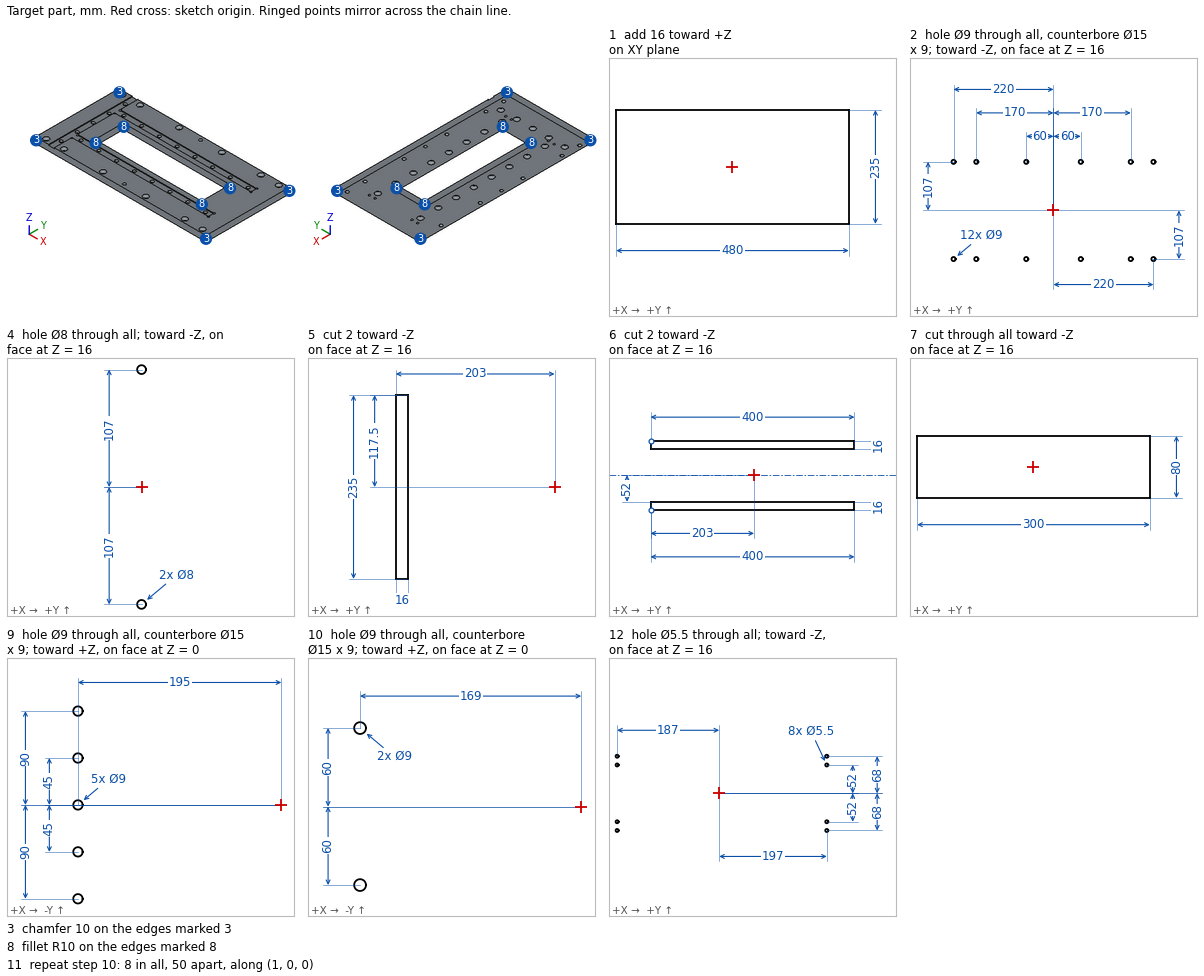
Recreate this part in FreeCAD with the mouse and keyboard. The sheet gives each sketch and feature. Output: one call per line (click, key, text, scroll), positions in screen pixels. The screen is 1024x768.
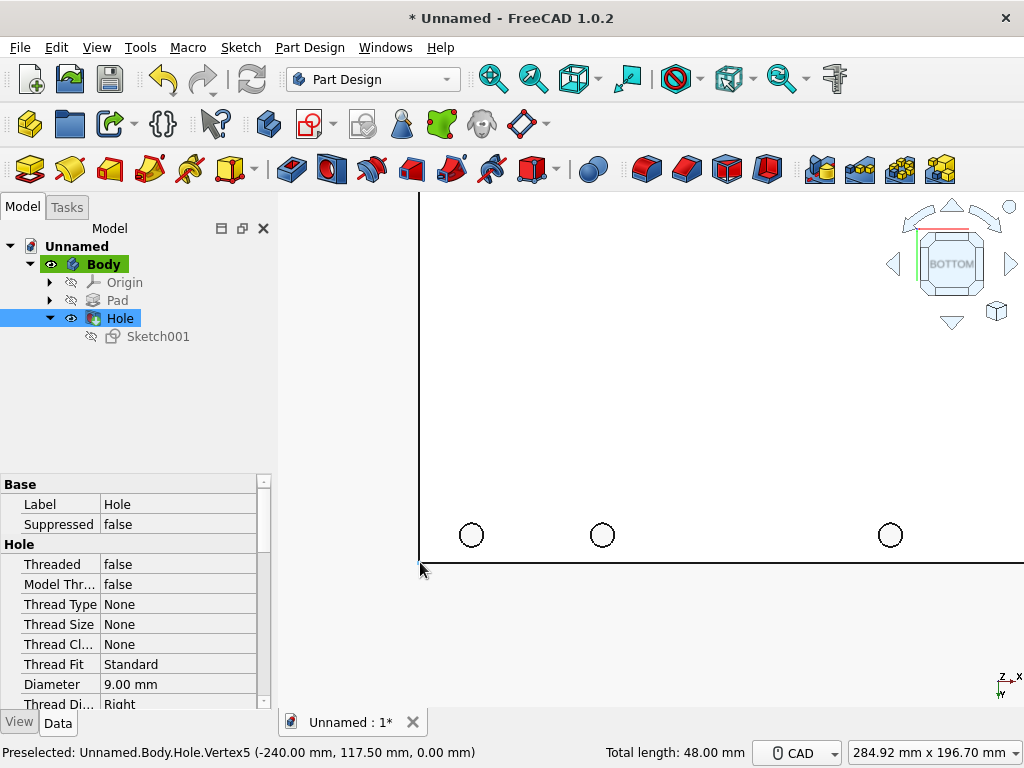
click(494, 80)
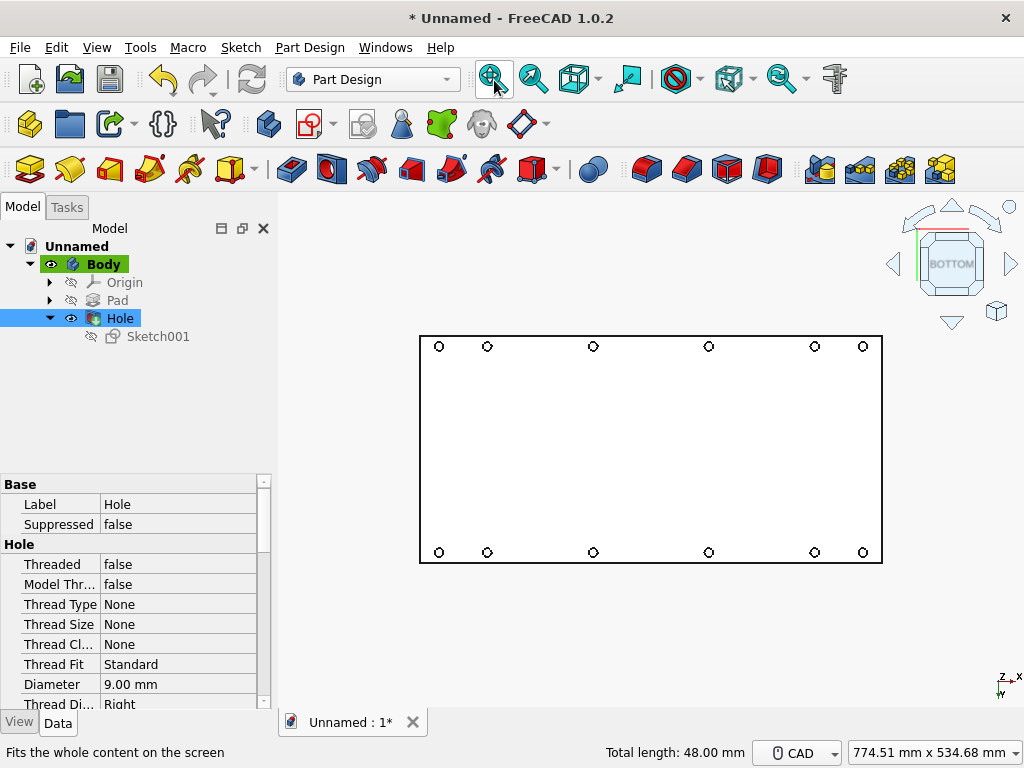
key(4)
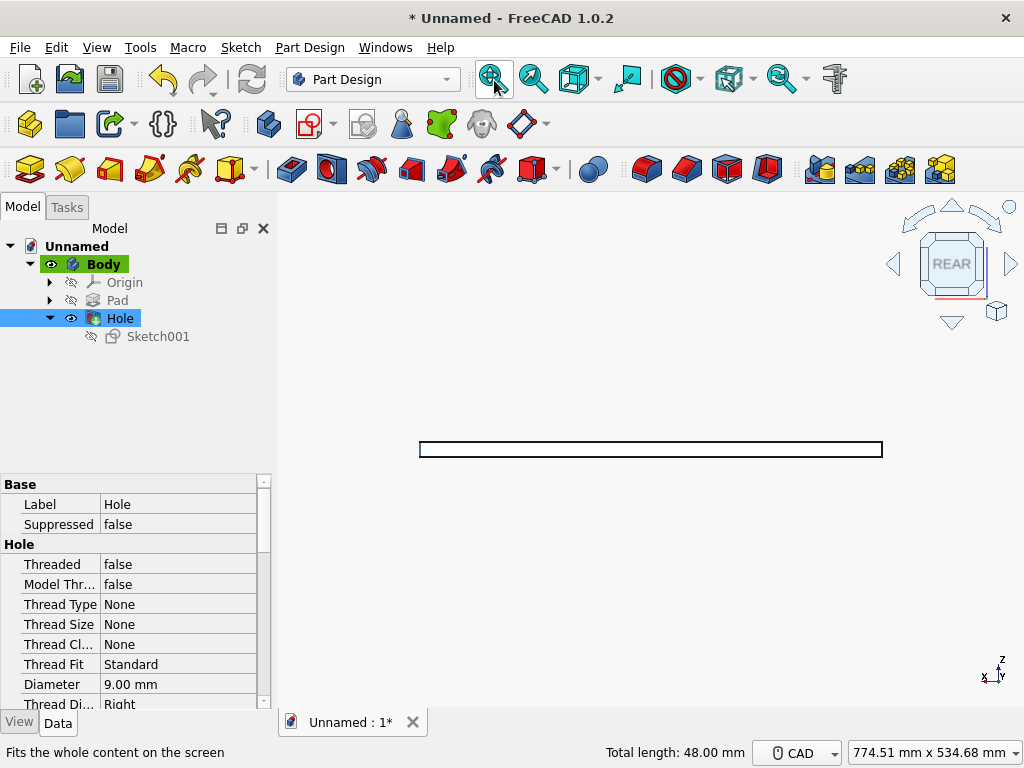
click(882, 449, ctrl)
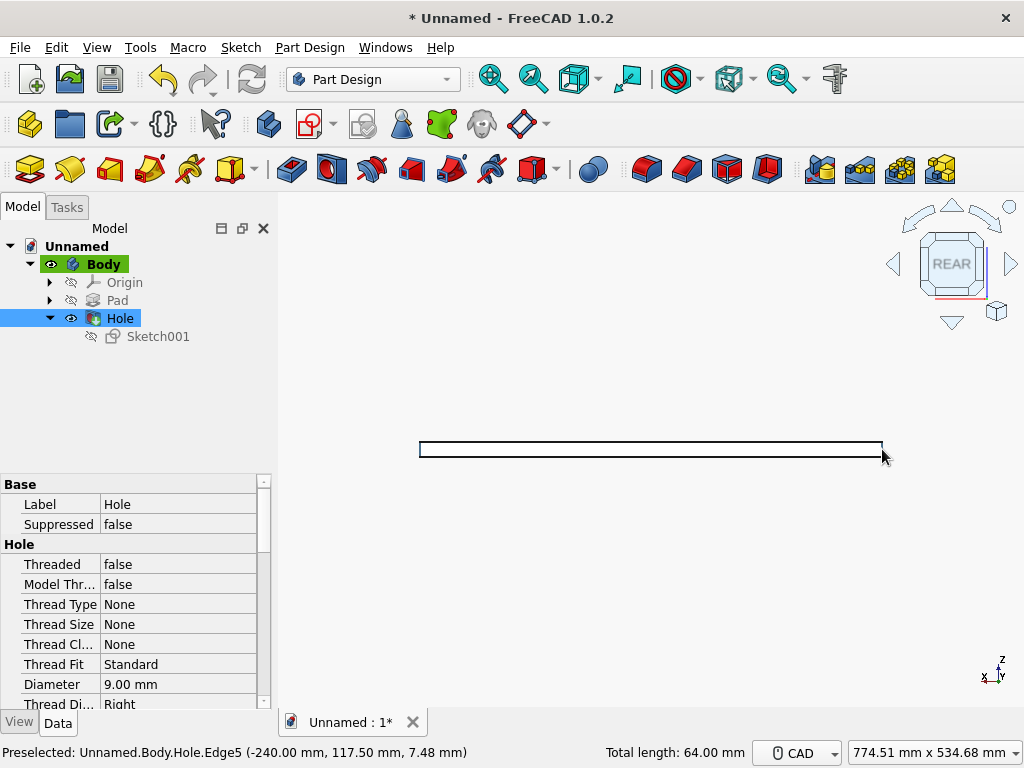
click(688, 170)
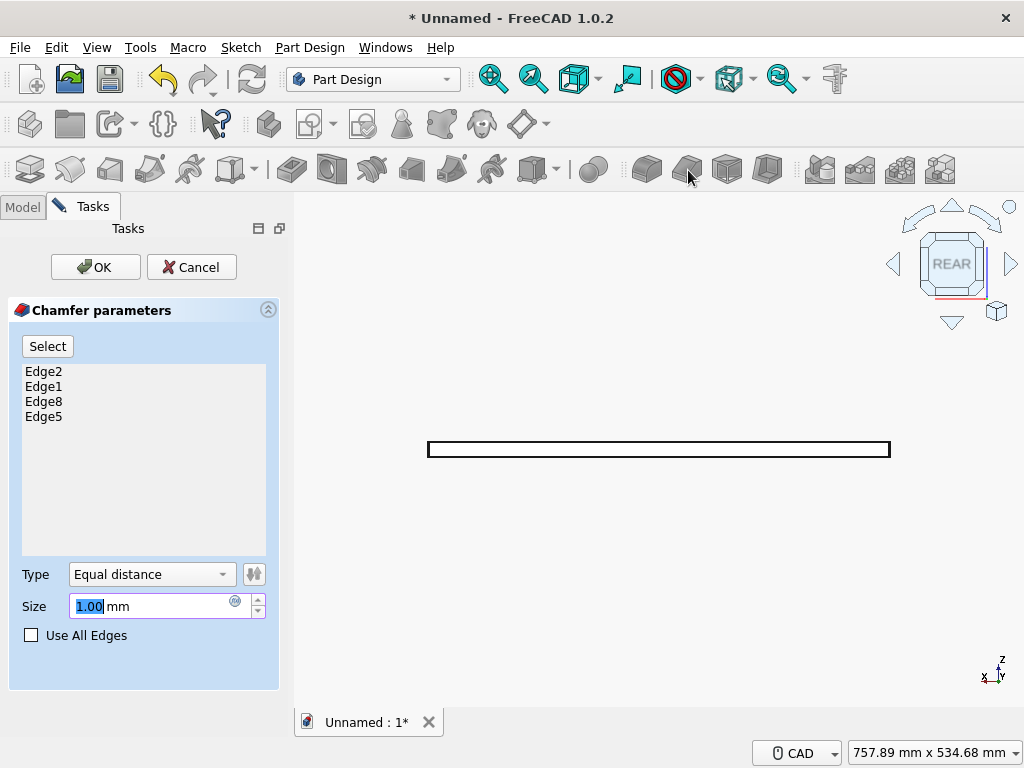
text(10)
key(Tab)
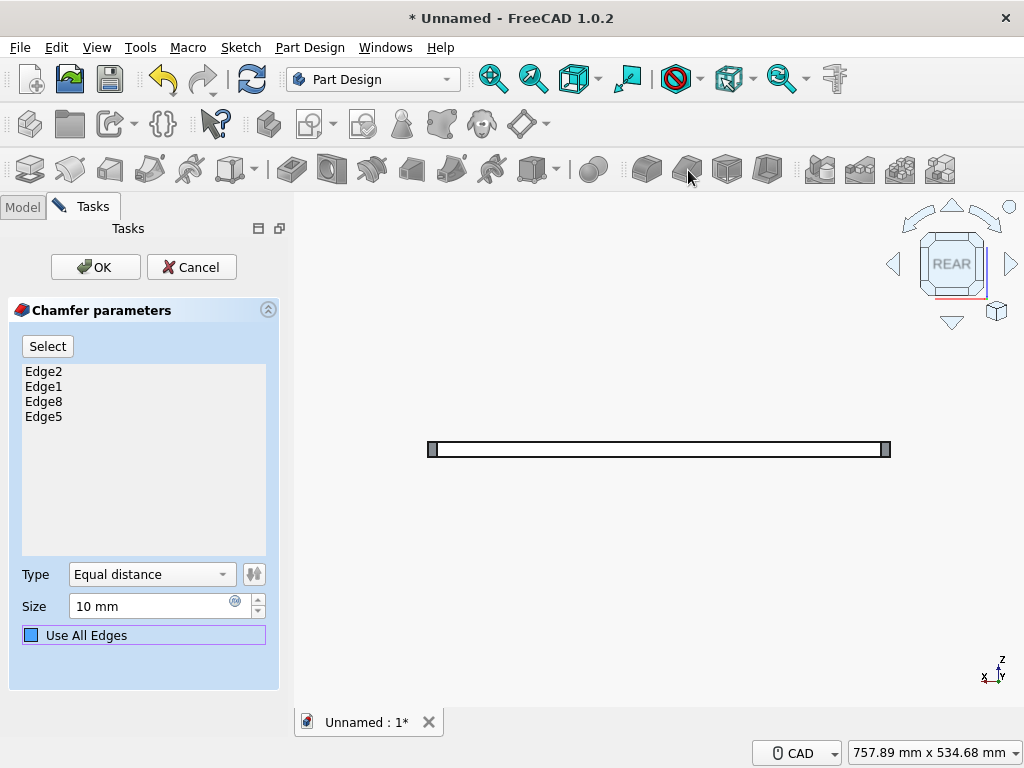
click(96, 267)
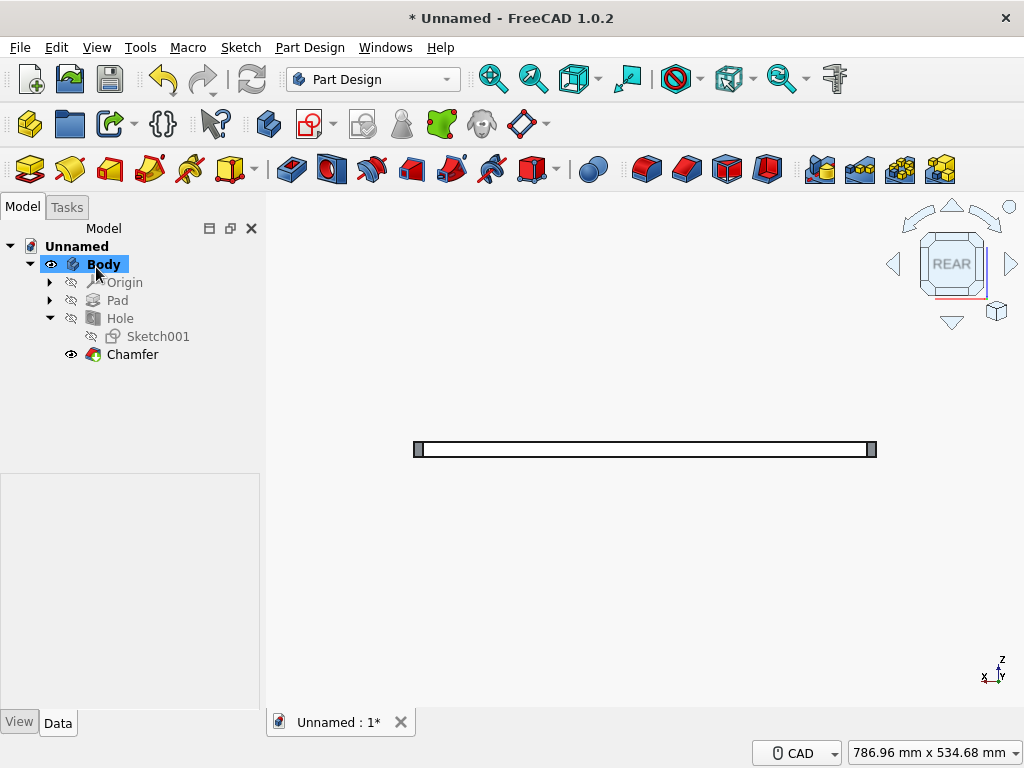
key(0)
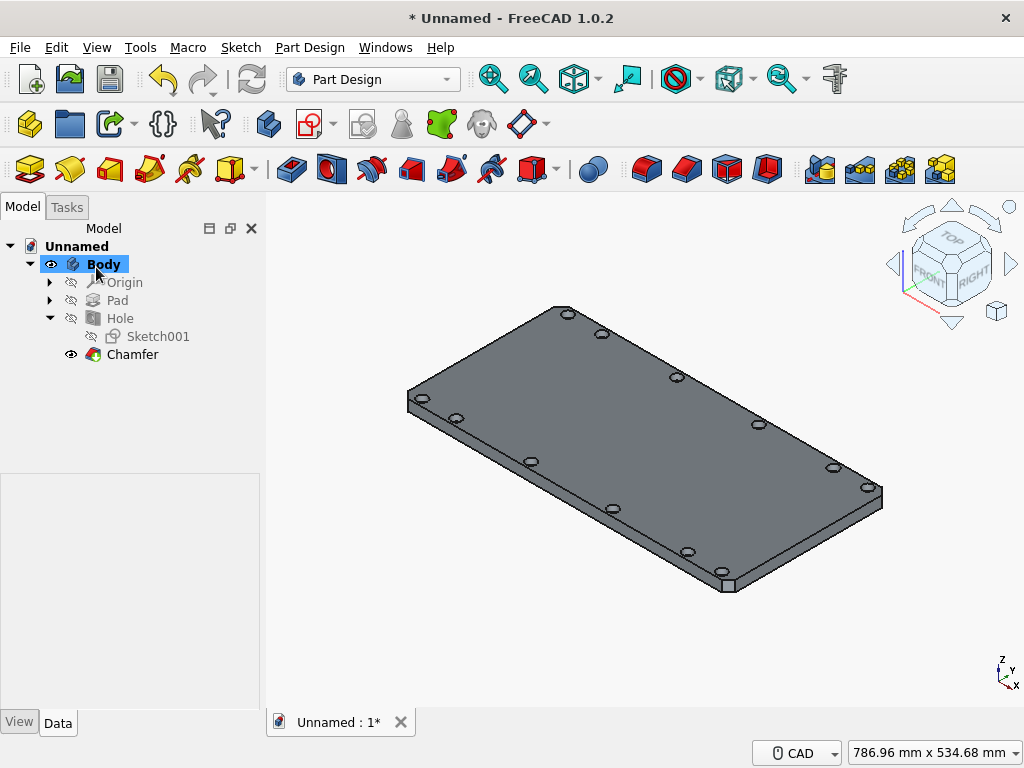
click(645, 442)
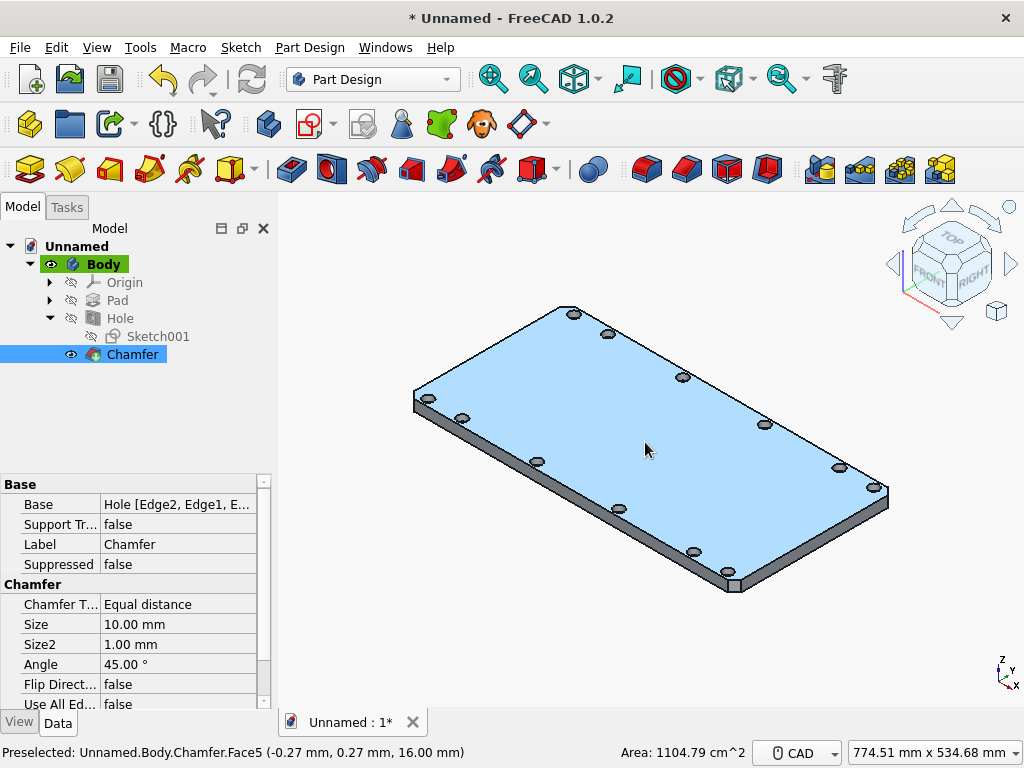
click(310, 124)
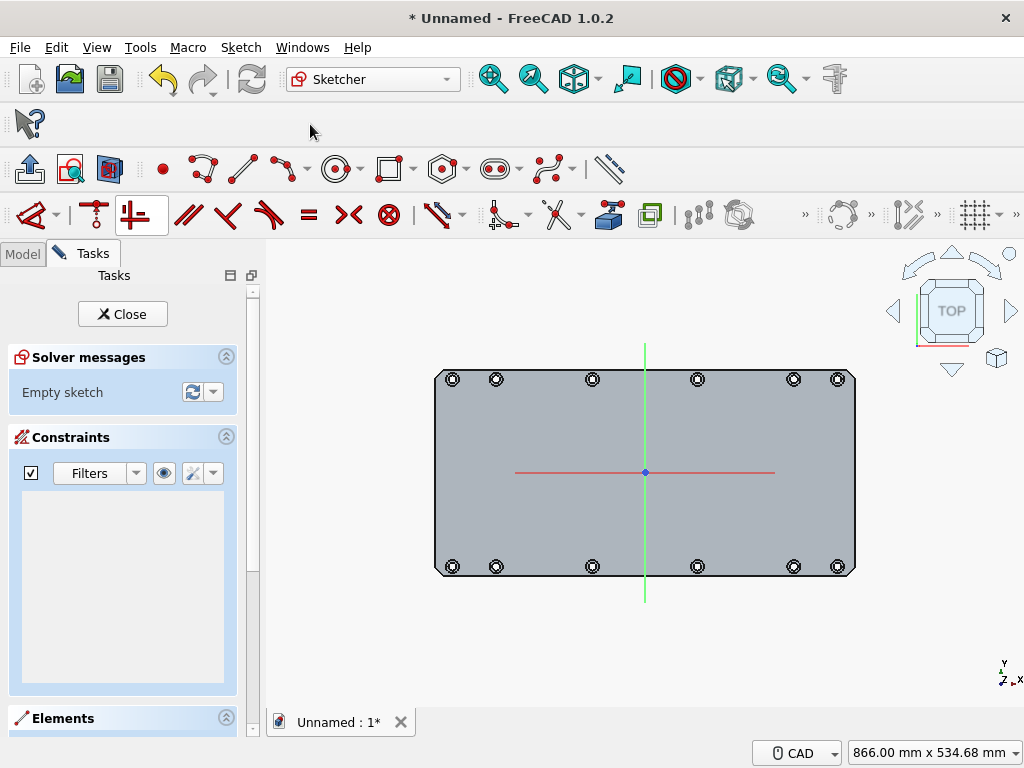
scroll(784, 473, up, 2)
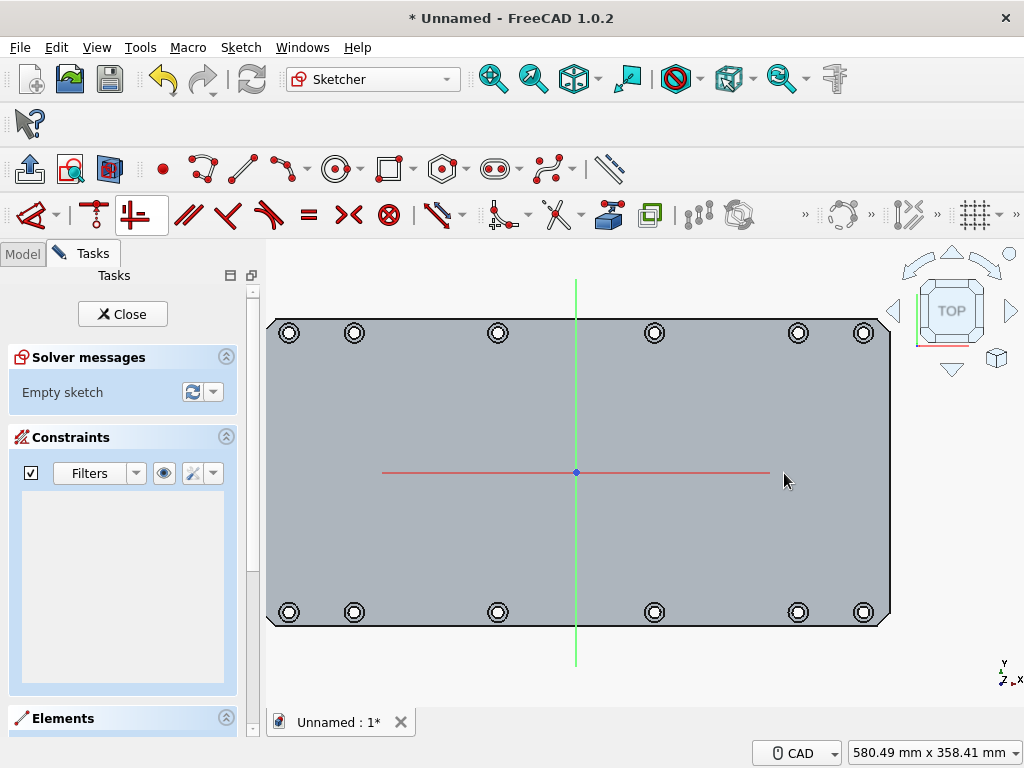
click(336, 170)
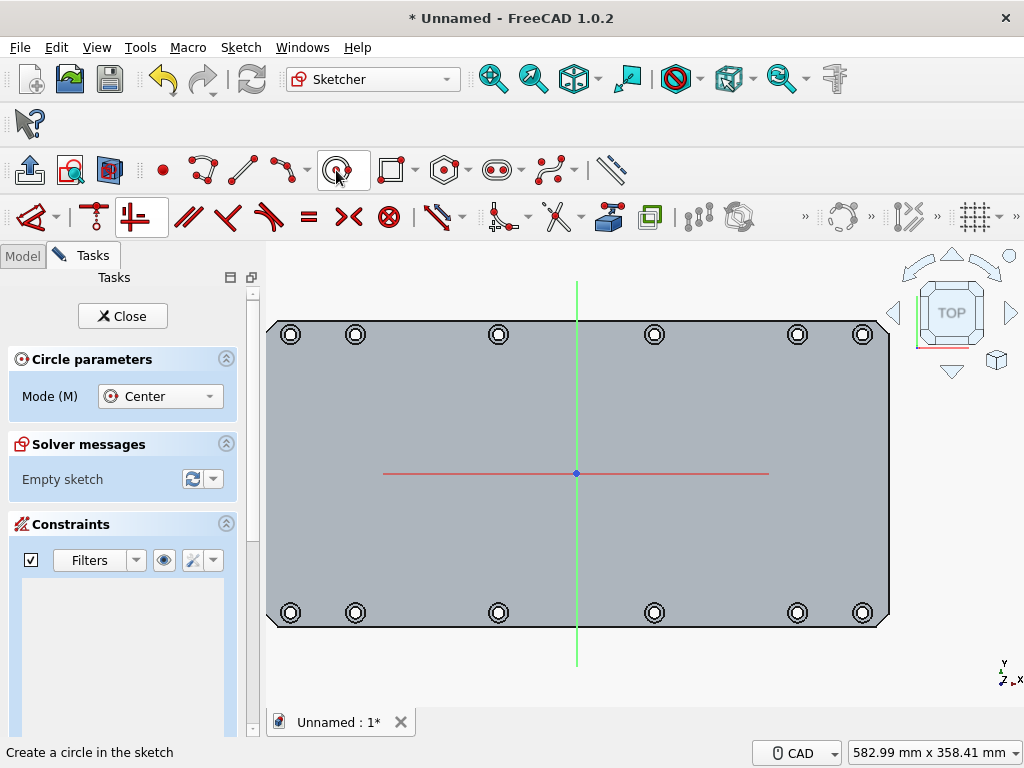
scroll(577, 613, up, 8)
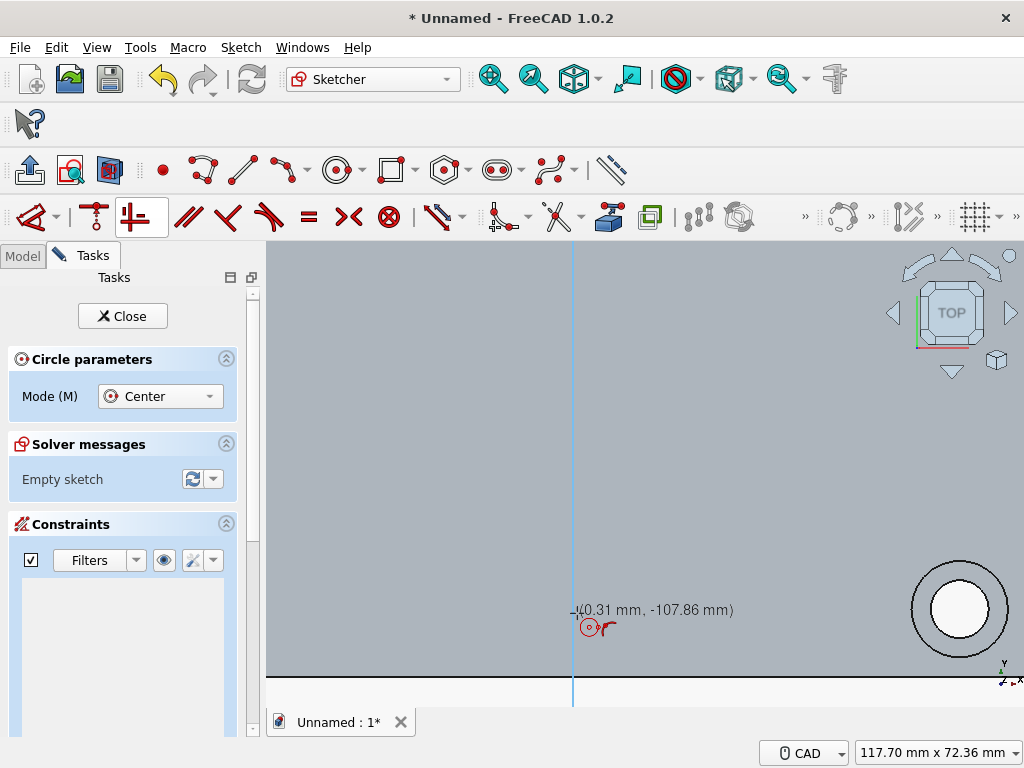
scroll(577, 614, down, 8)